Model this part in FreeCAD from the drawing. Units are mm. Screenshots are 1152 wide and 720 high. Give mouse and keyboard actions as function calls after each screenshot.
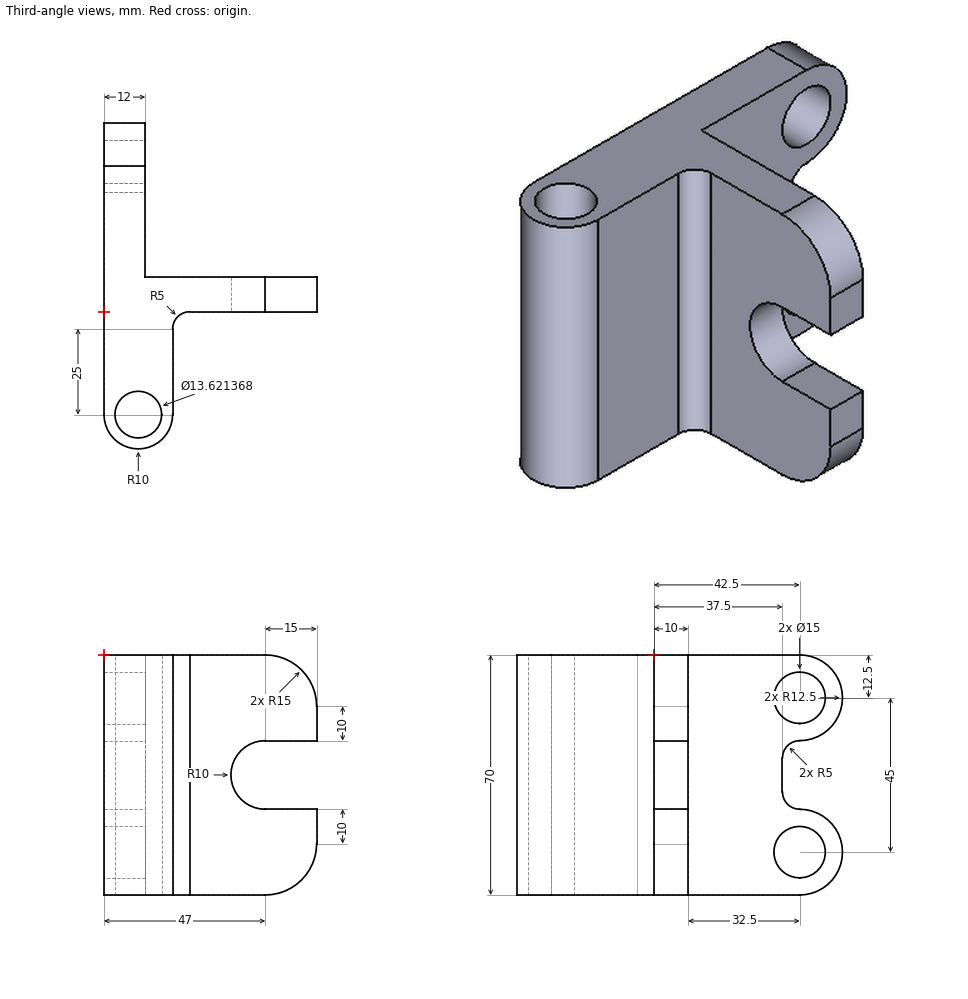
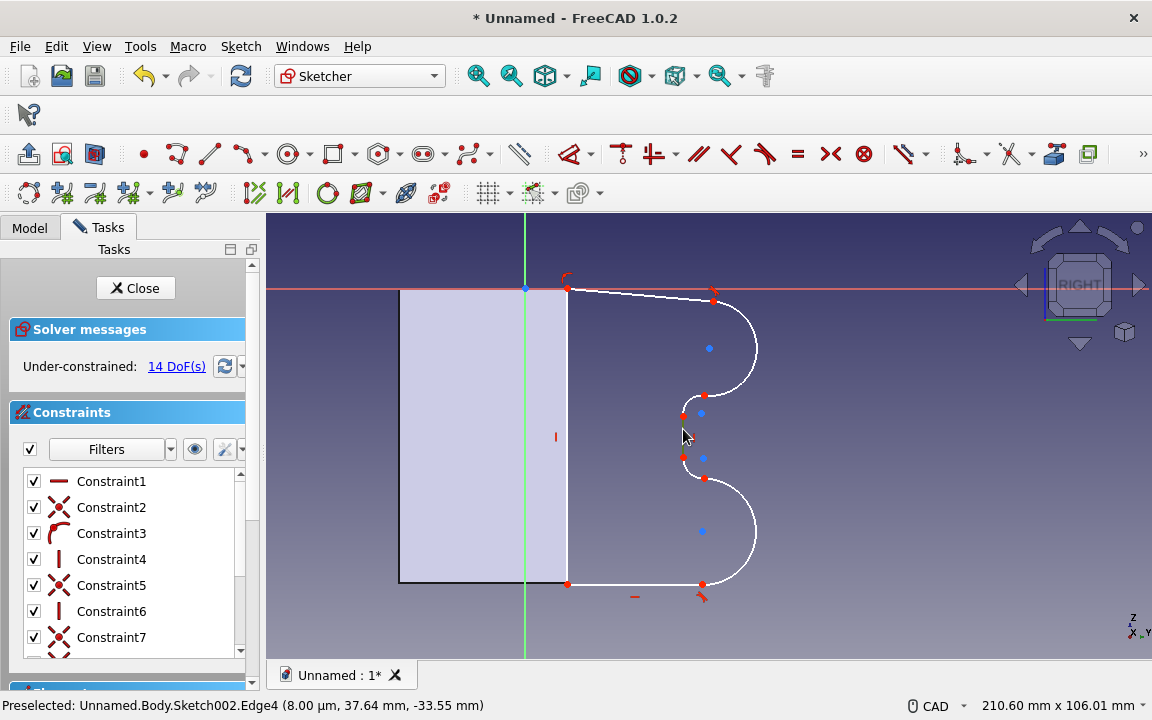
scroll(694, 397, up, 2)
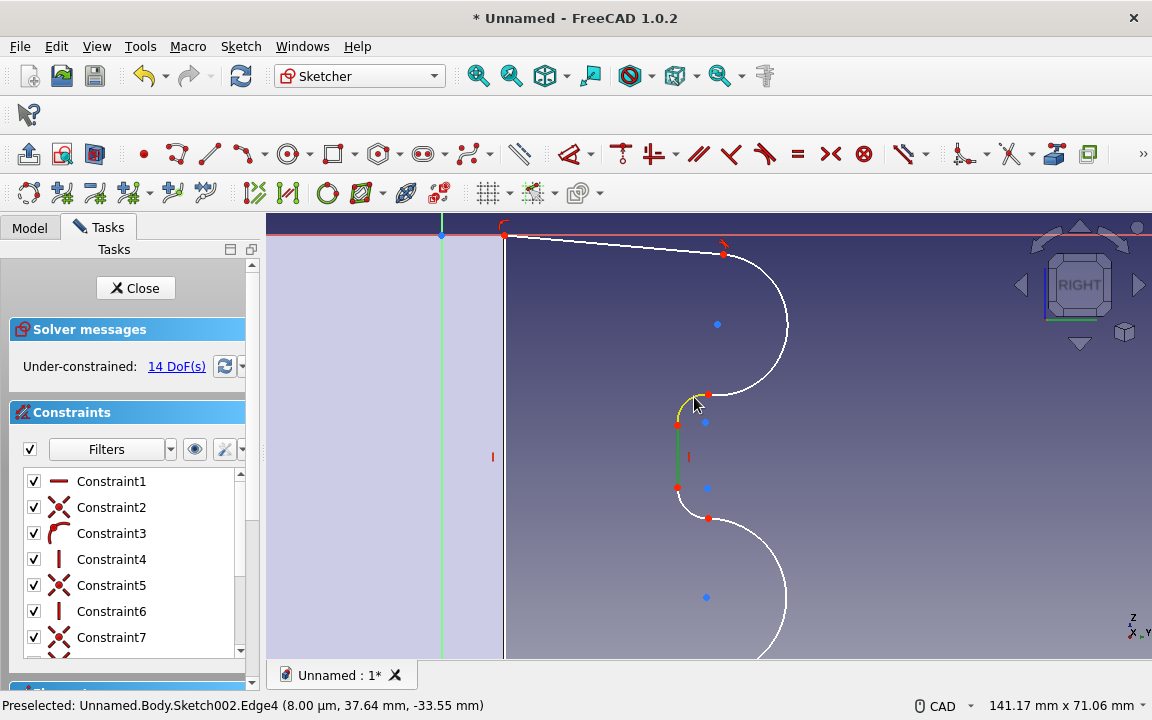
click(694, 397)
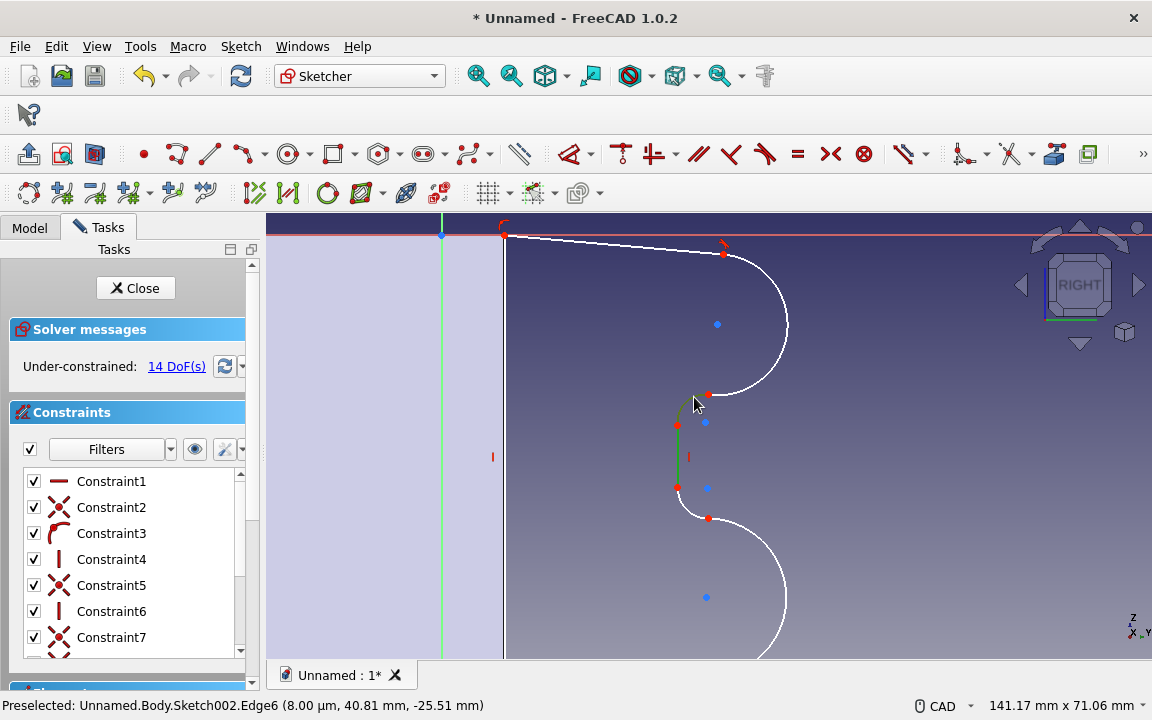
click(765, 154)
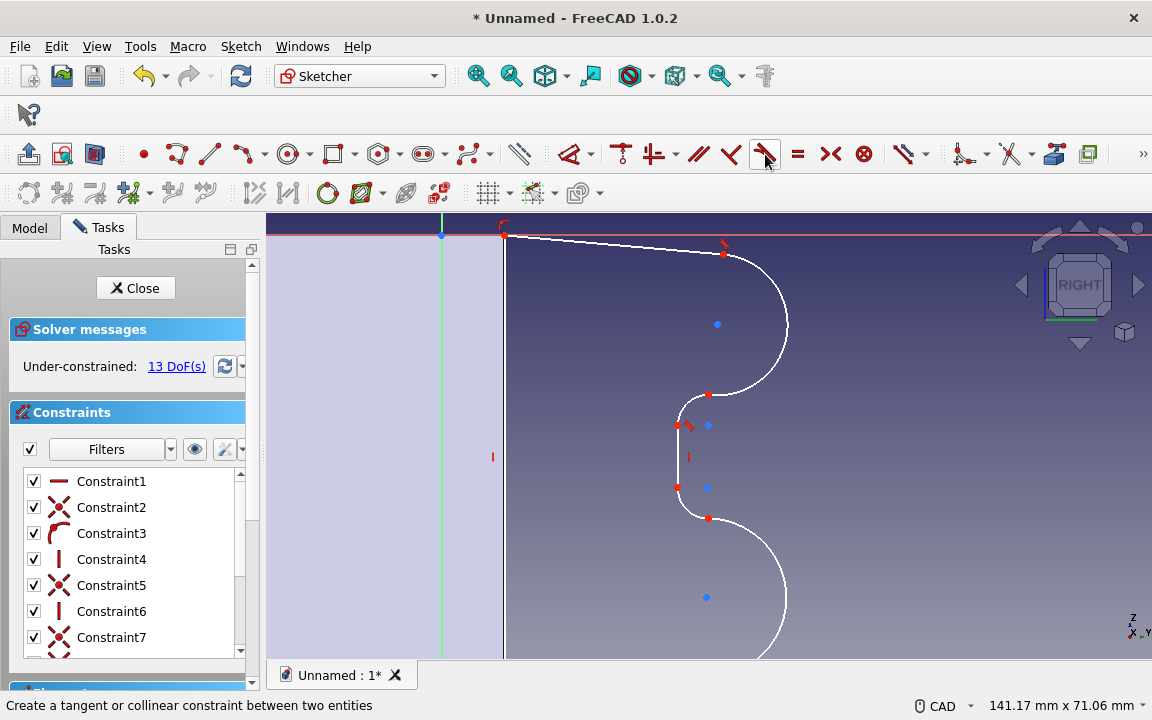
click(678, 444)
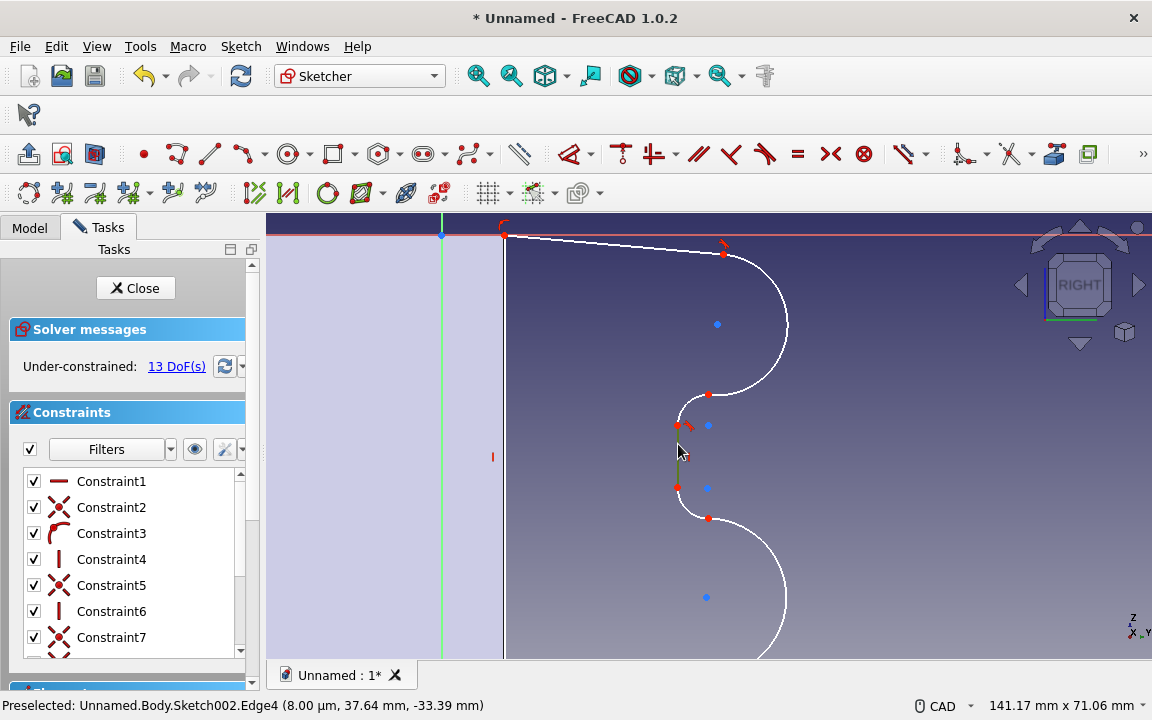
click(681, 502)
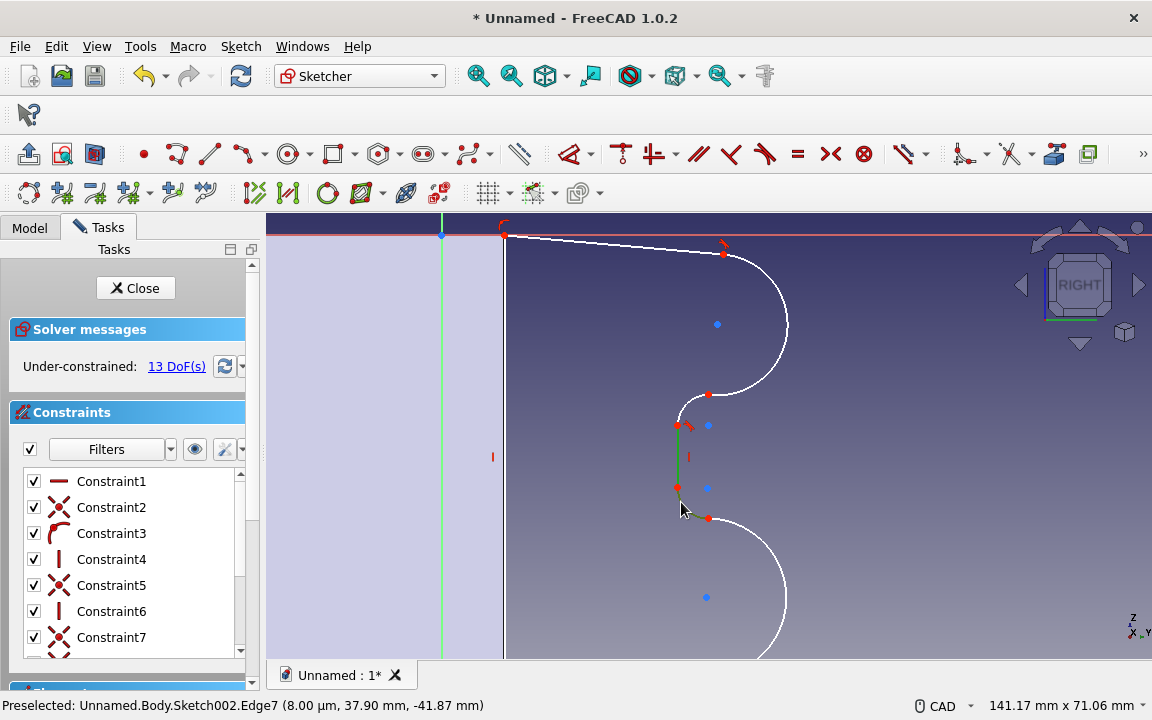
click(765, 154)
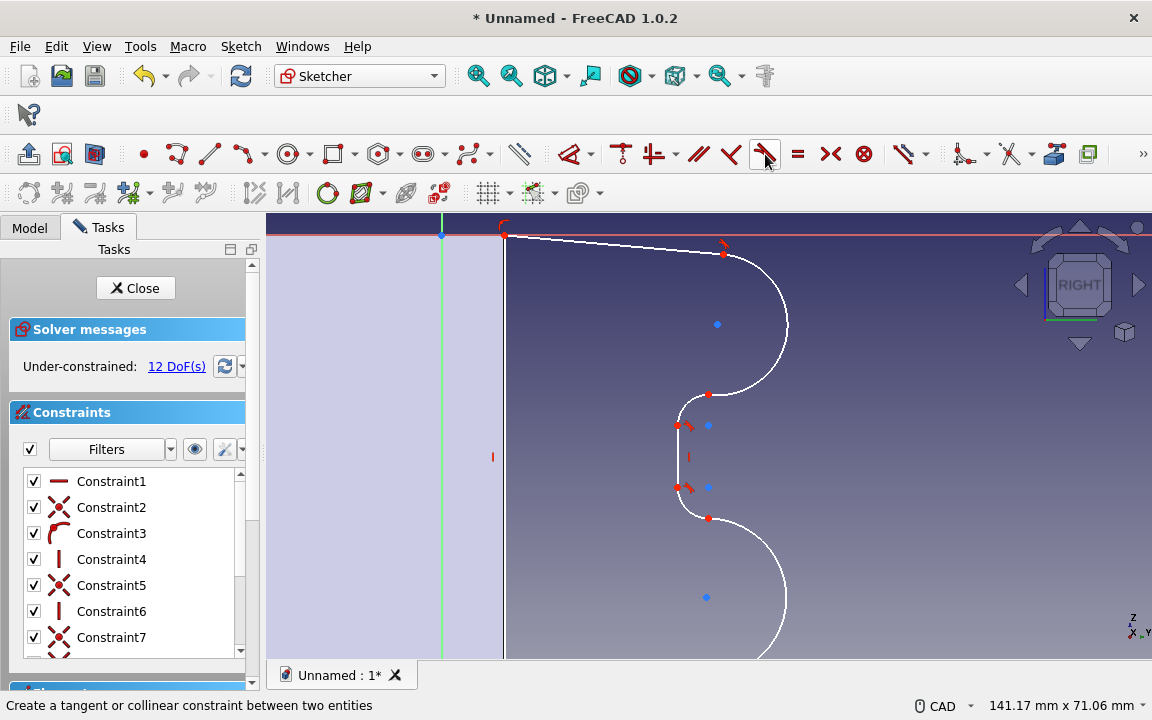
click(769, 372)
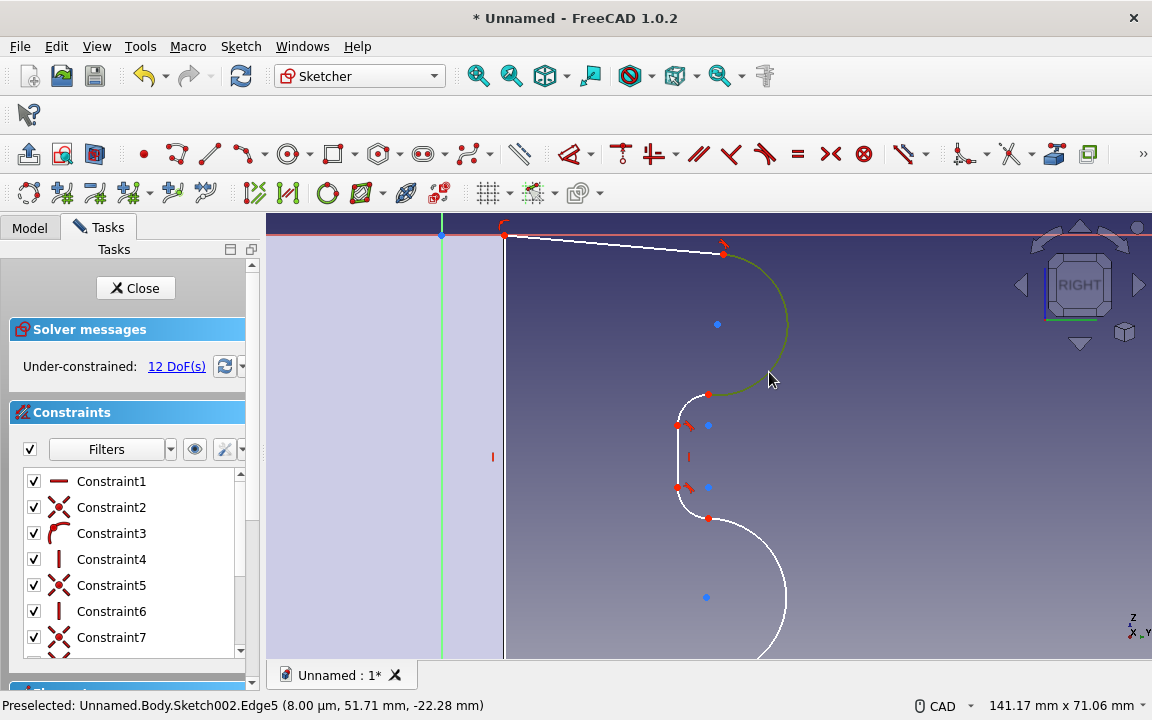
click(695, 398)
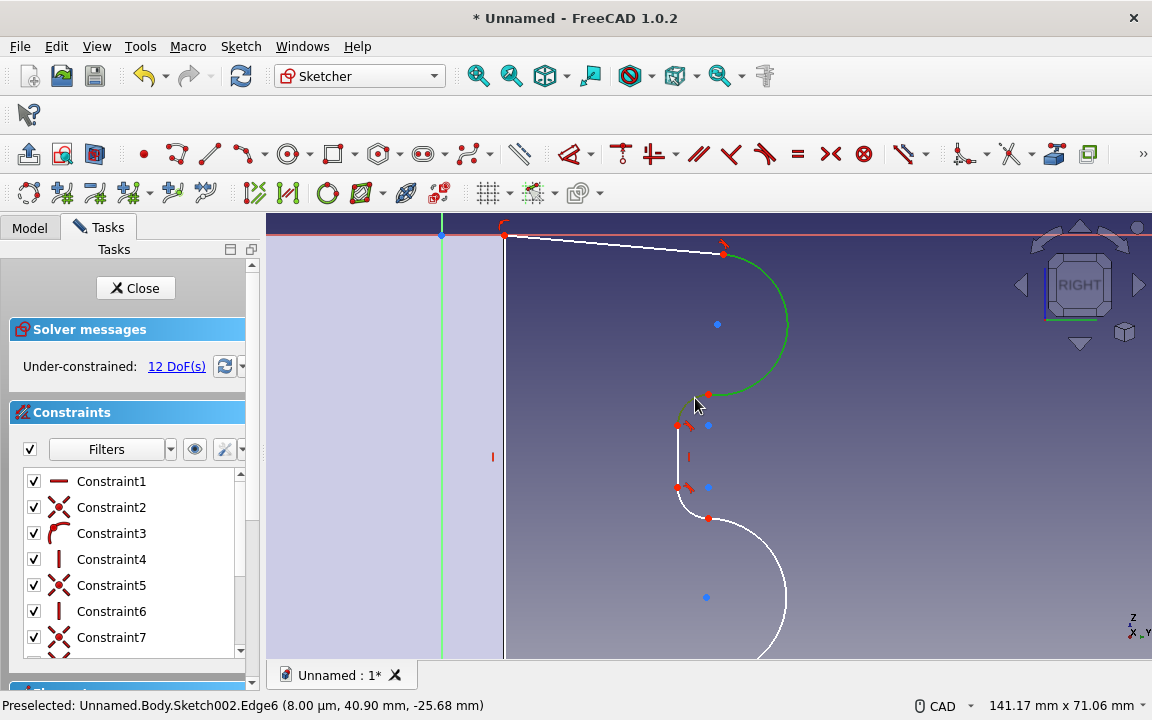
click(765, 154)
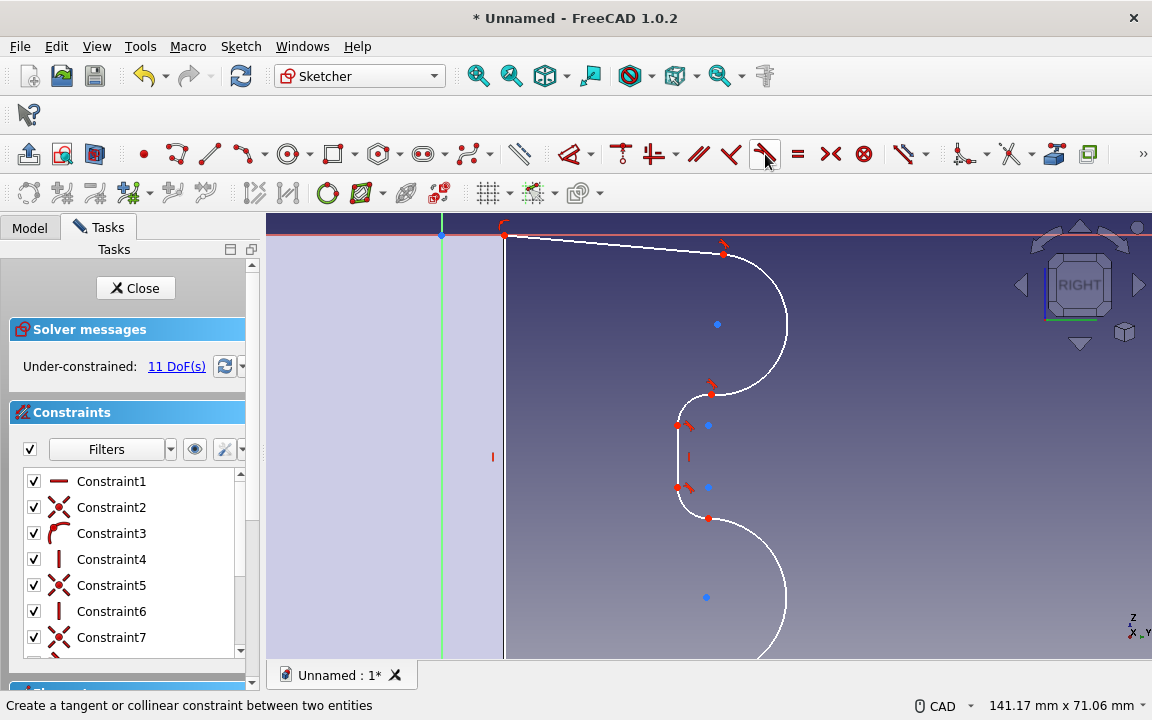
click(681, 502)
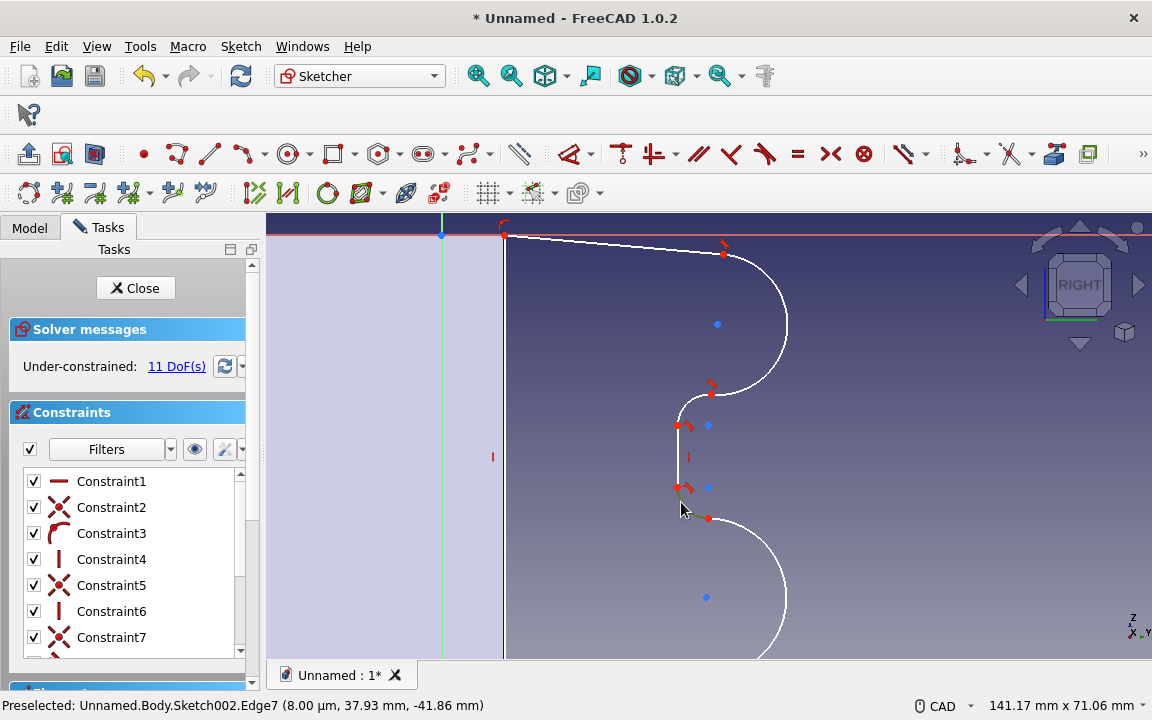
click(772, 552)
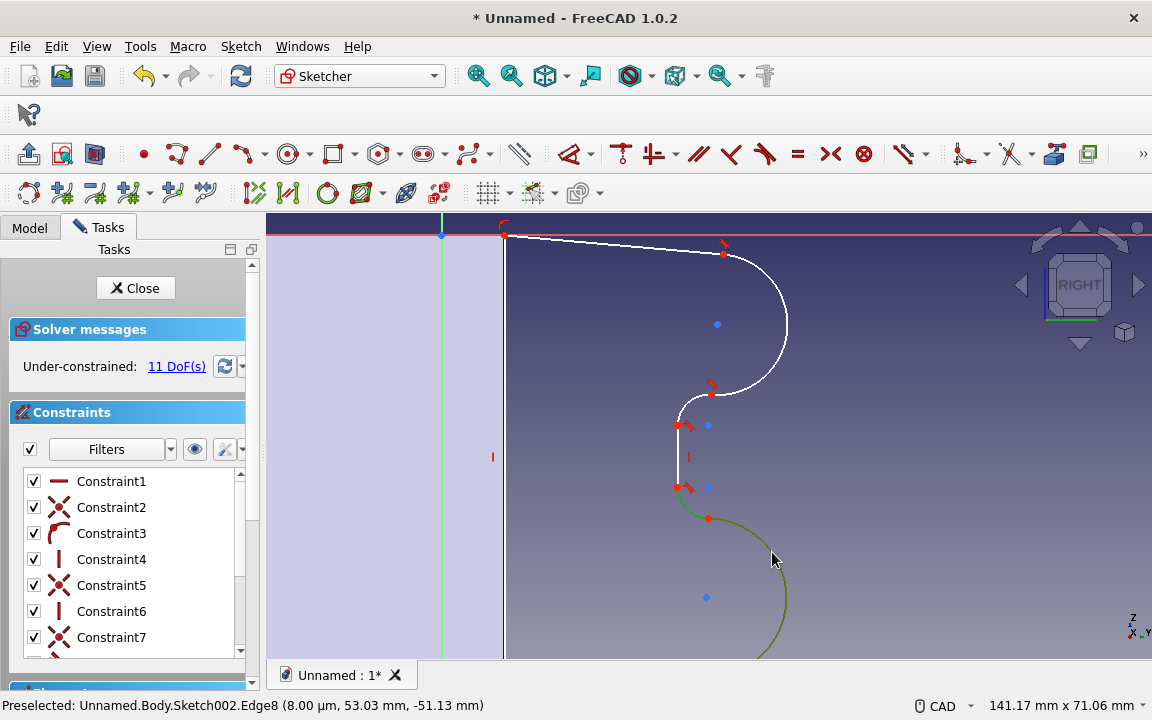
click(765, 154)